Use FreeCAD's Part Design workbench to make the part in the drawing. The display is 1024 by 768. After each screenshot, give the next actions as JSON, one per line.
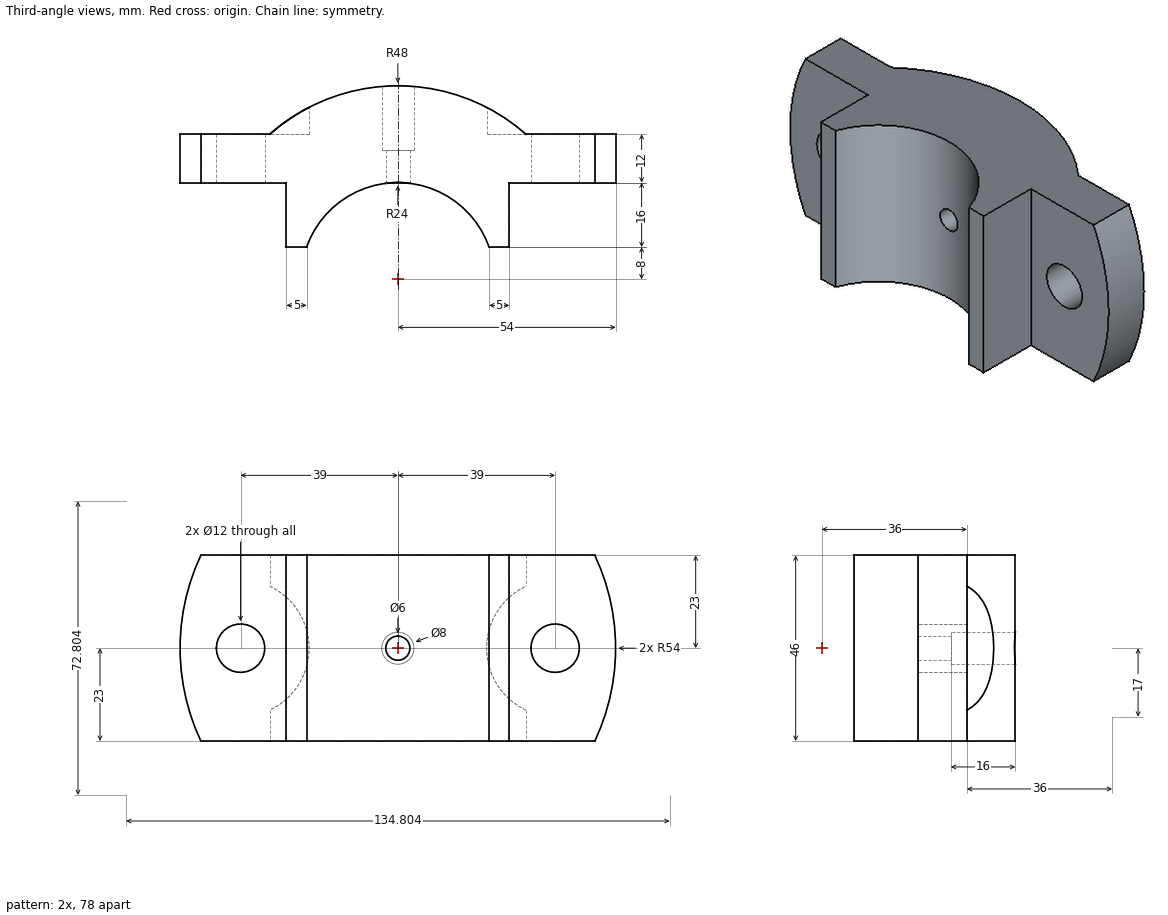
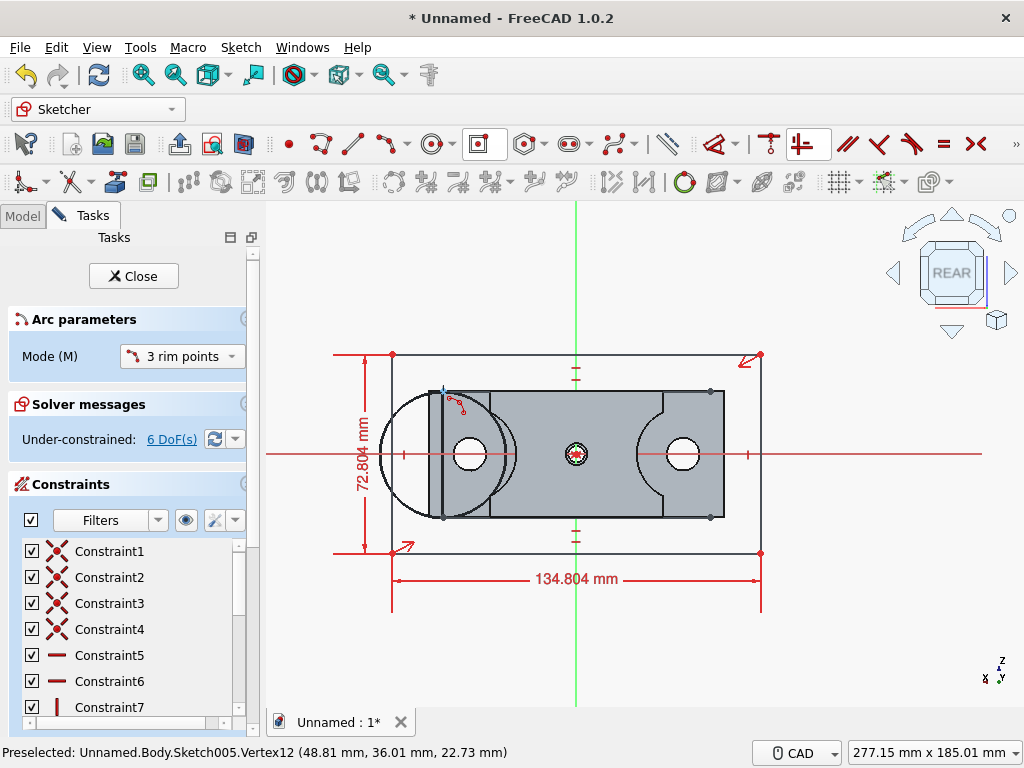
{"action": "scroll", "coordinate": [429, 441], "scroll_direction": "up", "scroll_amount": 2}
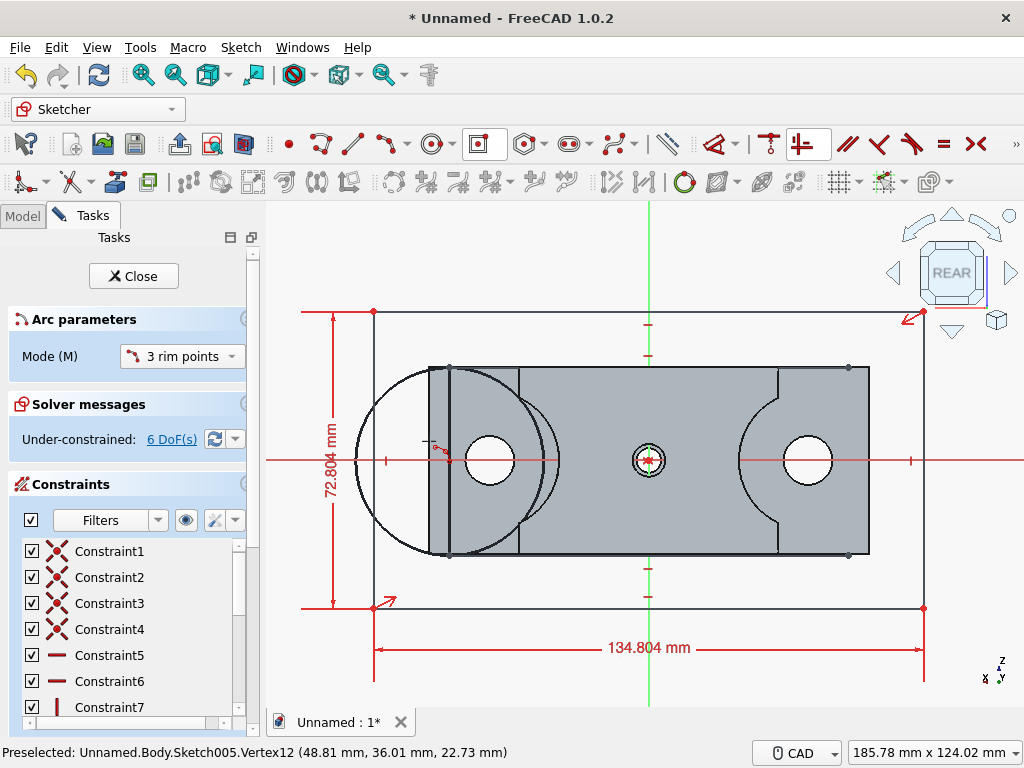
{"action": "left_click", "coordinate": [429, 441]}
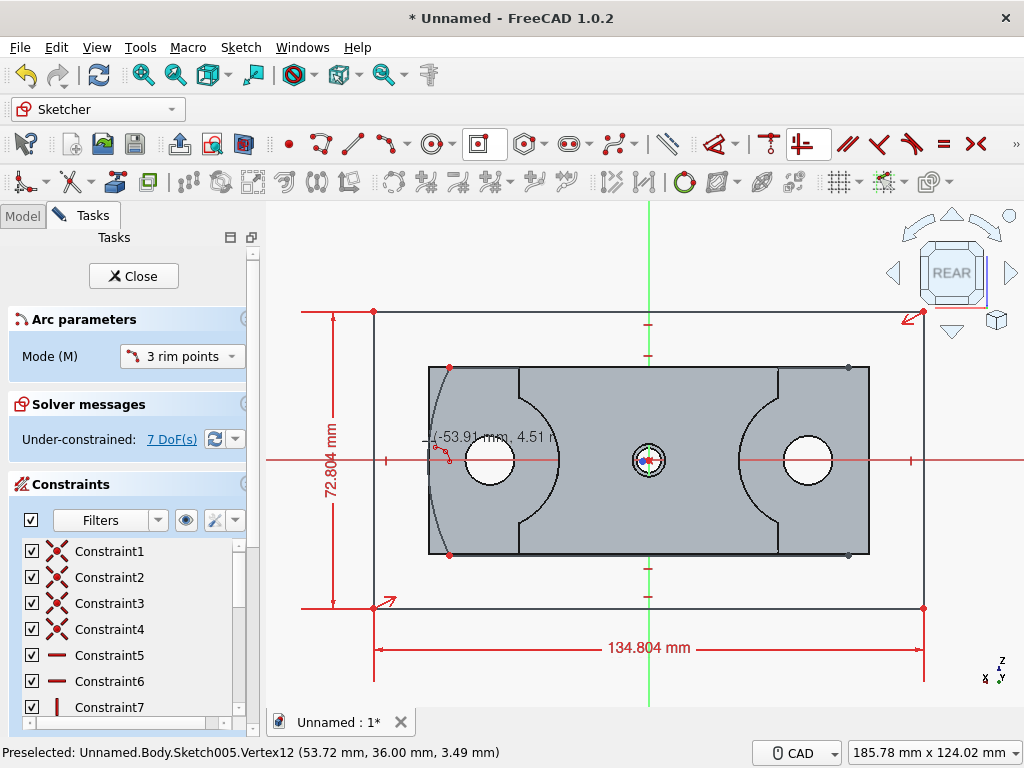
{"action": "left_click", "coordinate": [848, 368]}
{"action": "left_click", "coordinate": [848, 556]}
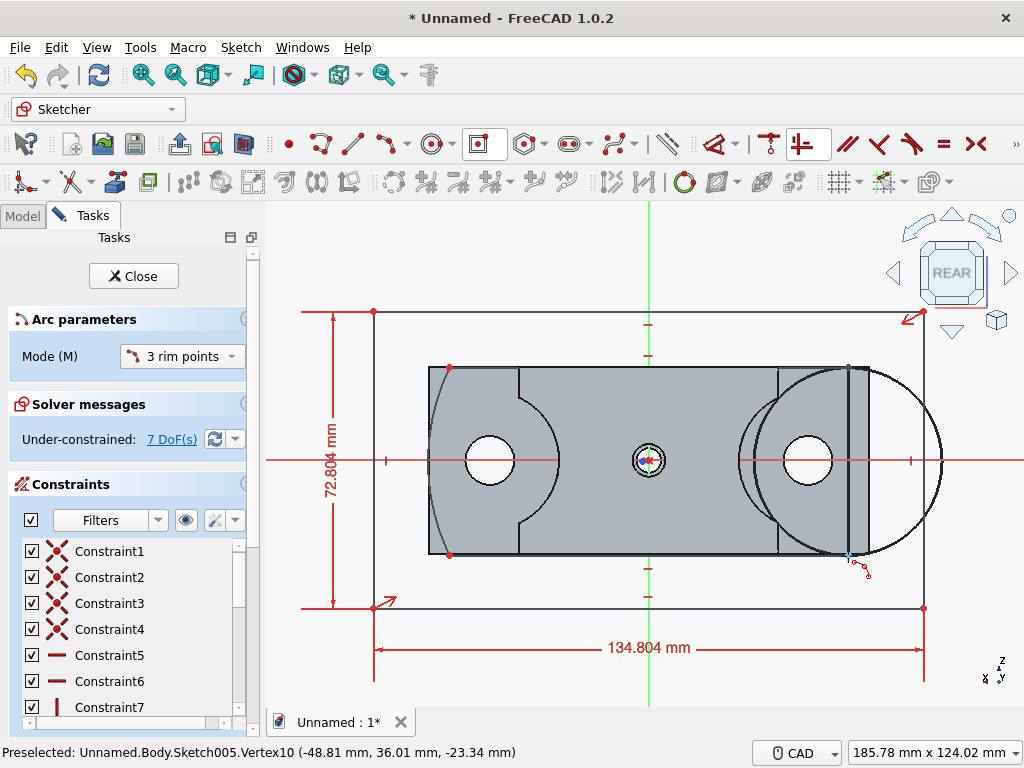
{"action": "scroll", "coordinate": [429, 441], "scroll_direction": "down", "scroll_amount": 2}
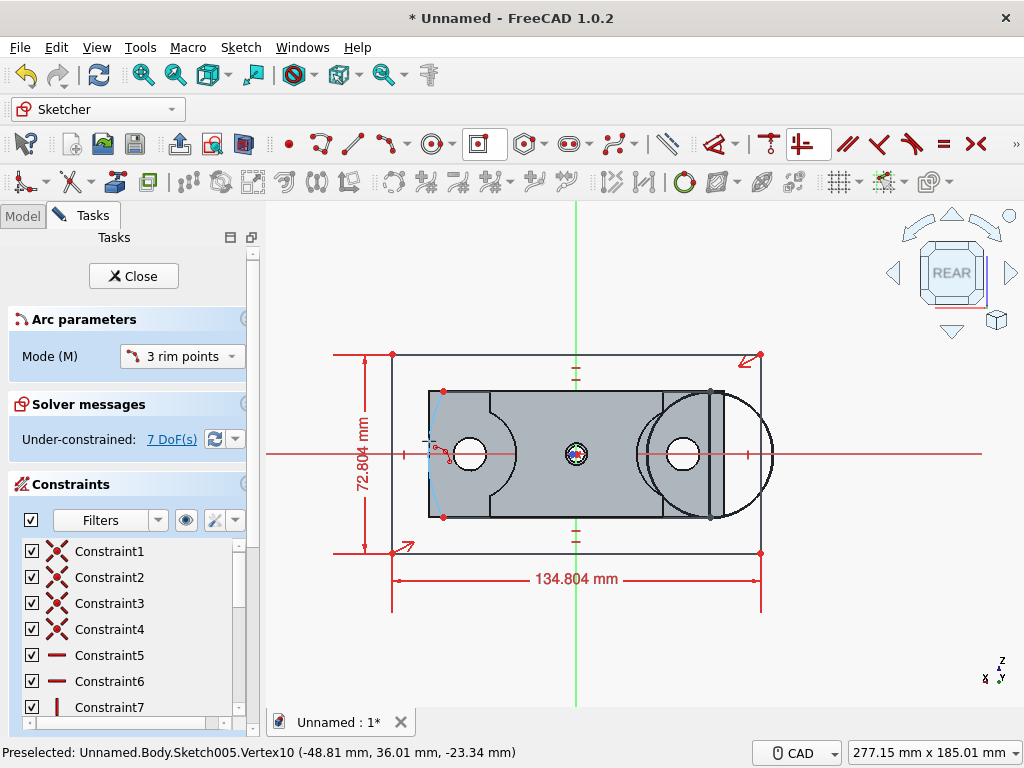
{"action": "scroll", "coordinate": [724, 467], "scroll_direction": "up", "scroll_amount": 2}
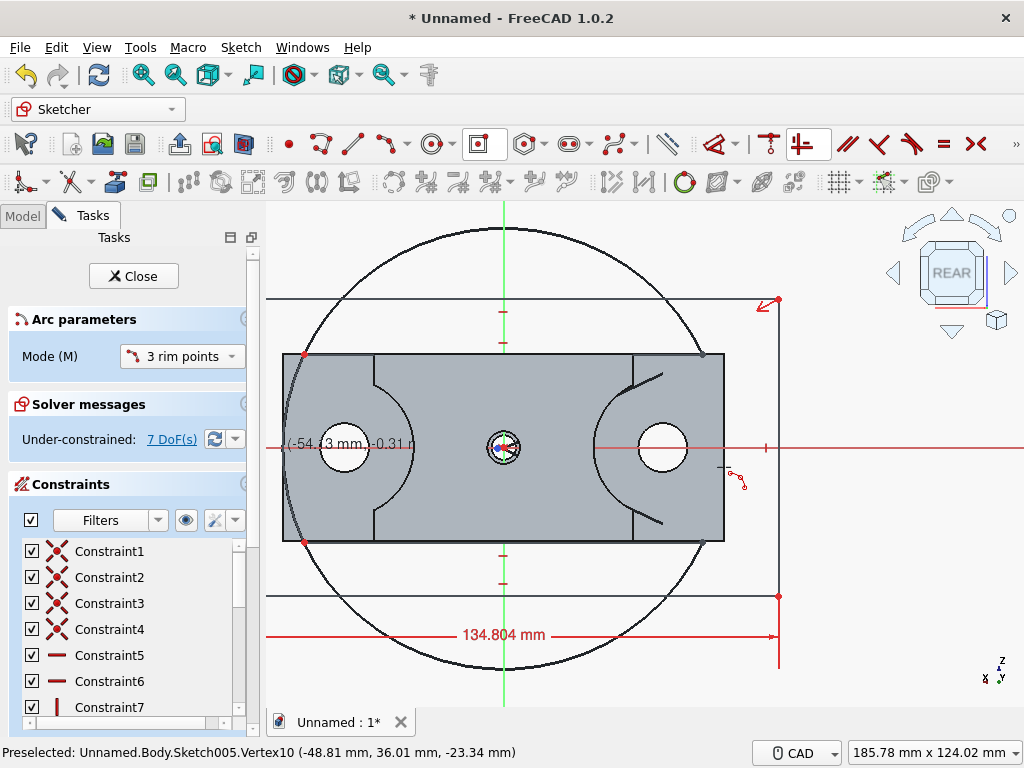
{"action": "left_click", "coordinate": [723, 467]}
{"action": "key", "text": "Escape"}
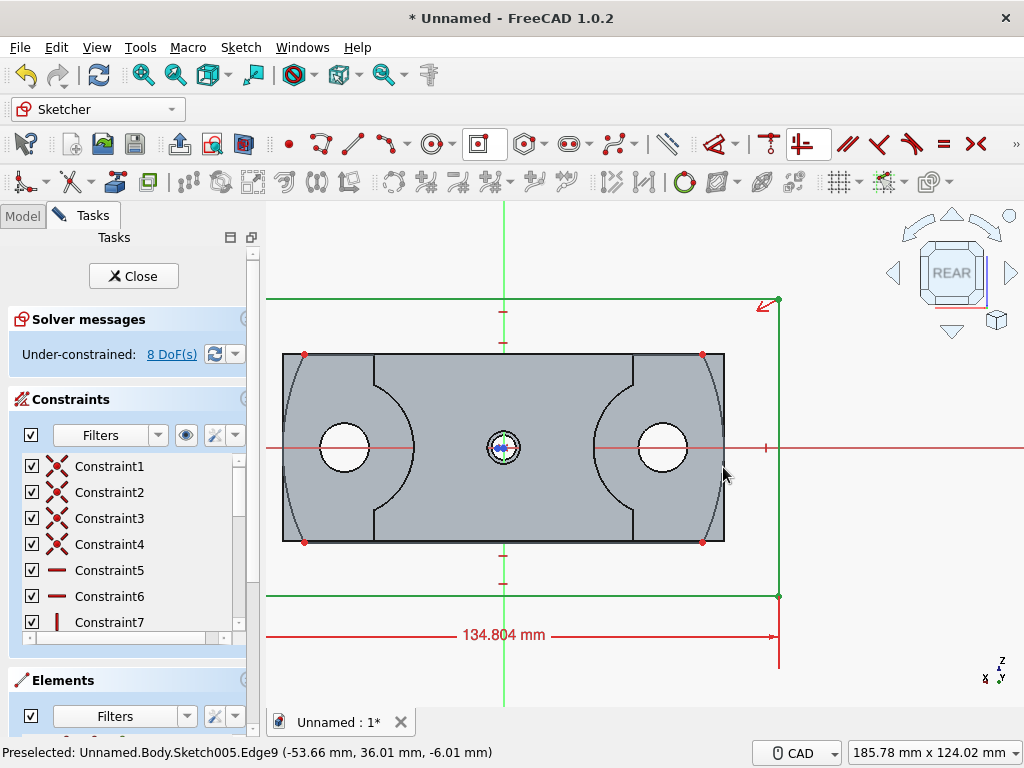
{"action": "scroll", "coordinate": [725, 467], "scroll_direction": "down", "scroll_amount": 2}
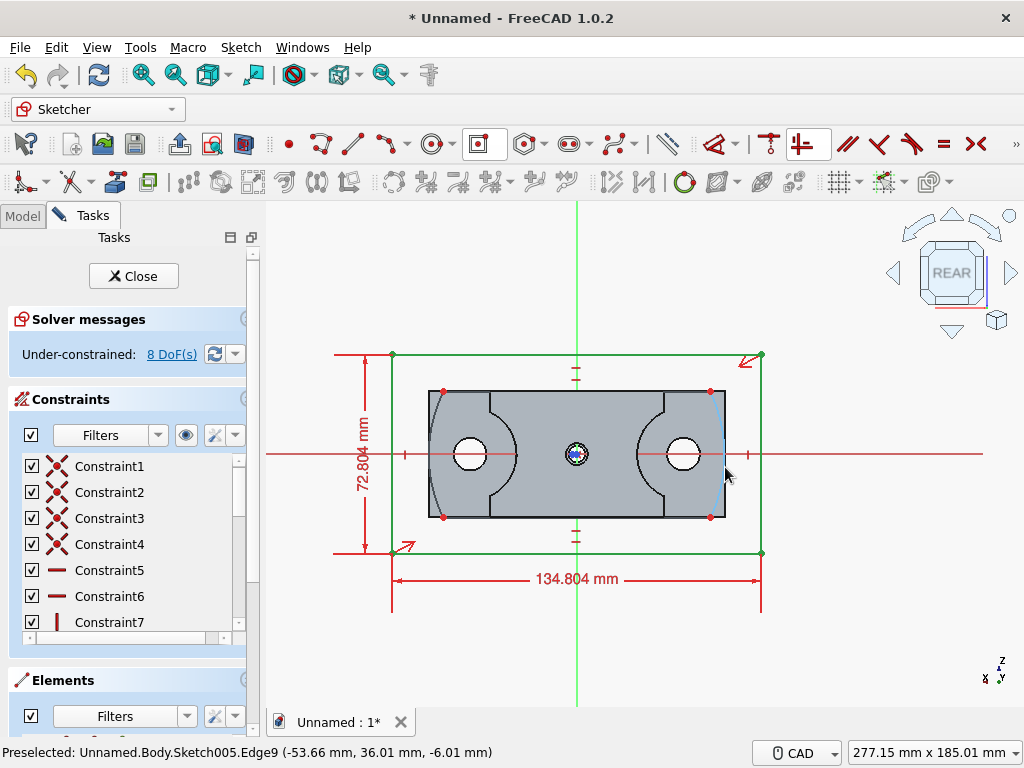
{"action": "left_click", "coordinate": [431, 429]}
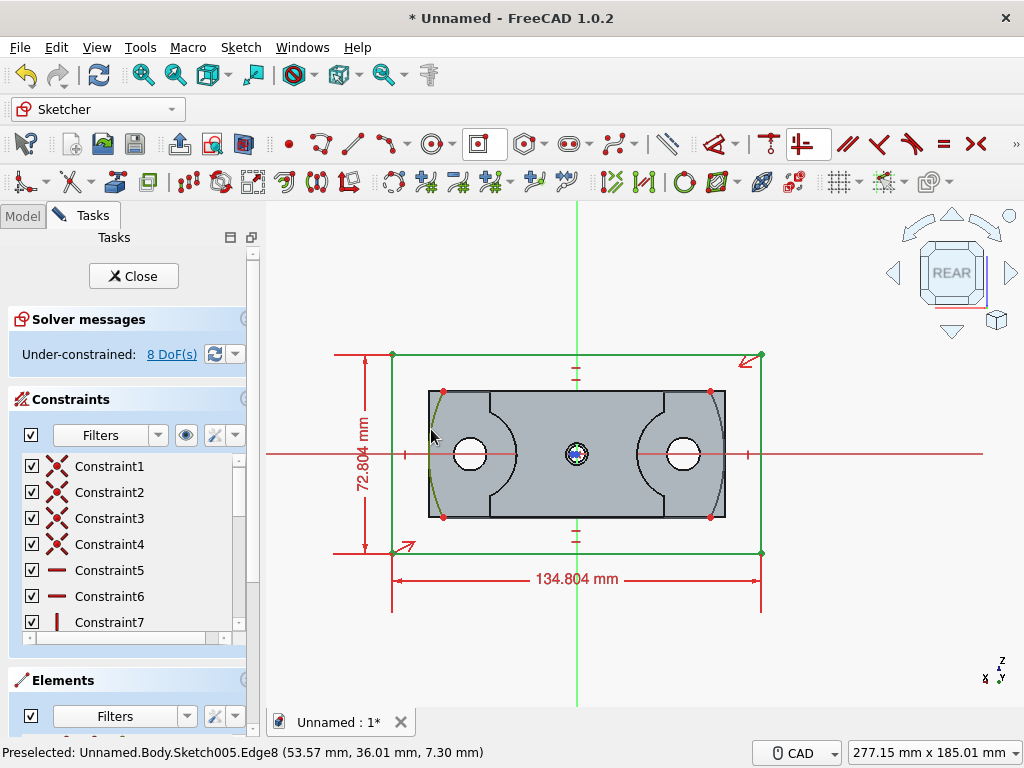
{"action": "left_click", "coordinate": [722, 481]}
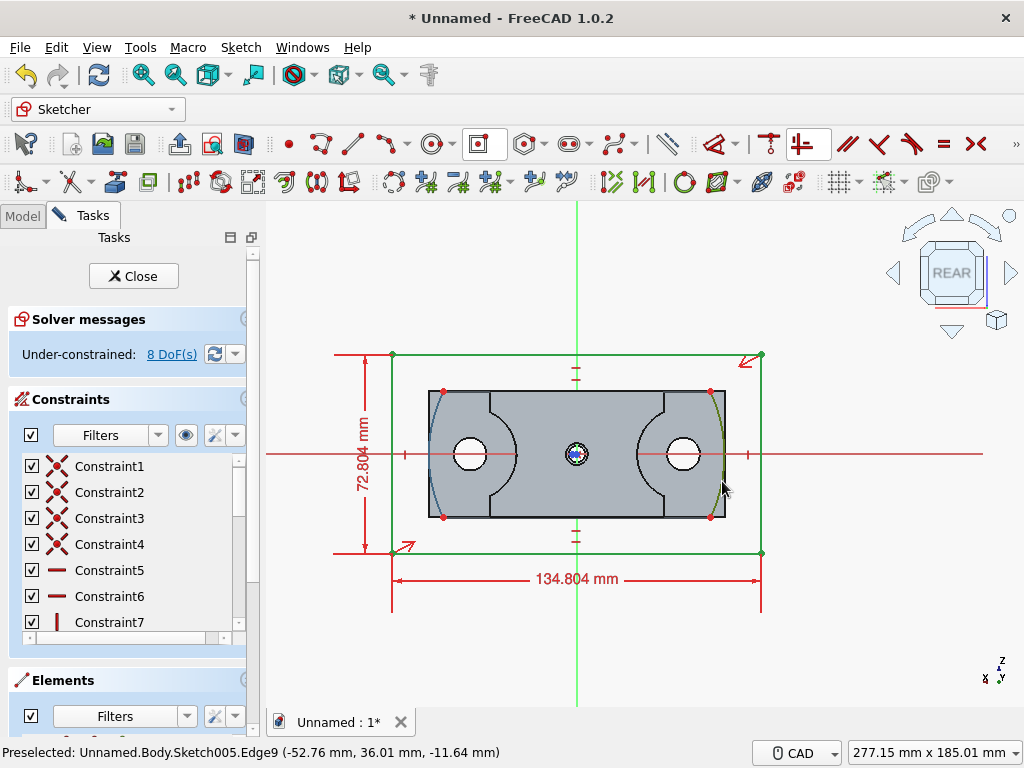
{"action": "left_click", "coordinate": [770, 144]}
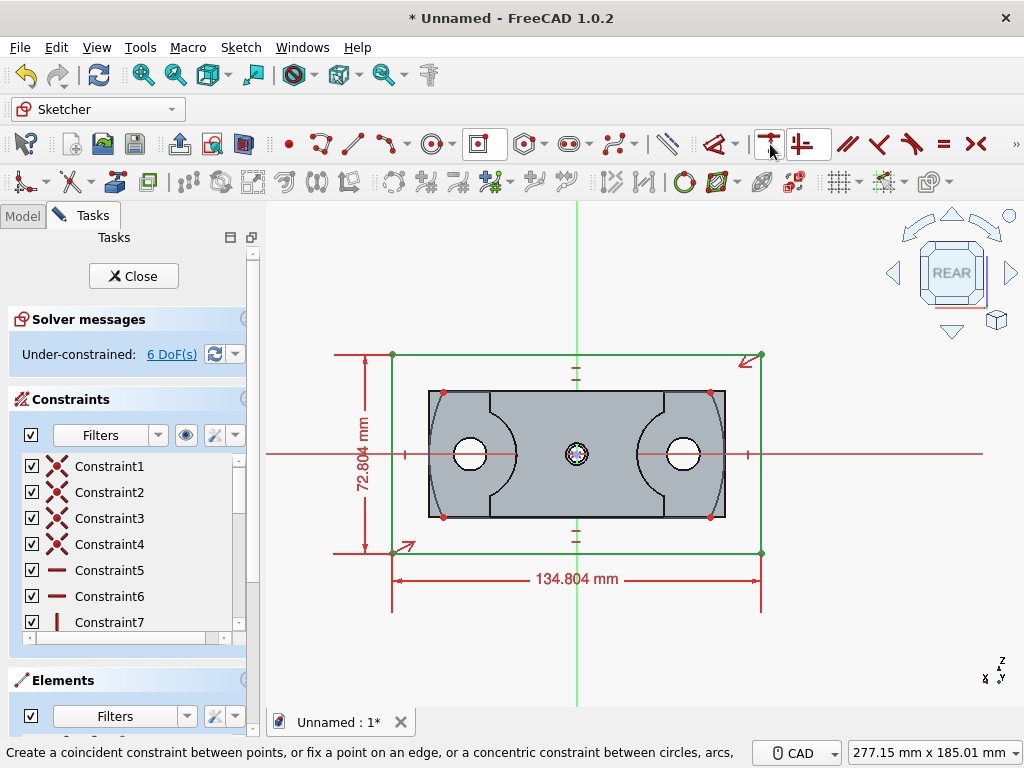
{"action": "left_click_drag", "start_coordinate": [566, 444], "coordinate": [587, 465]}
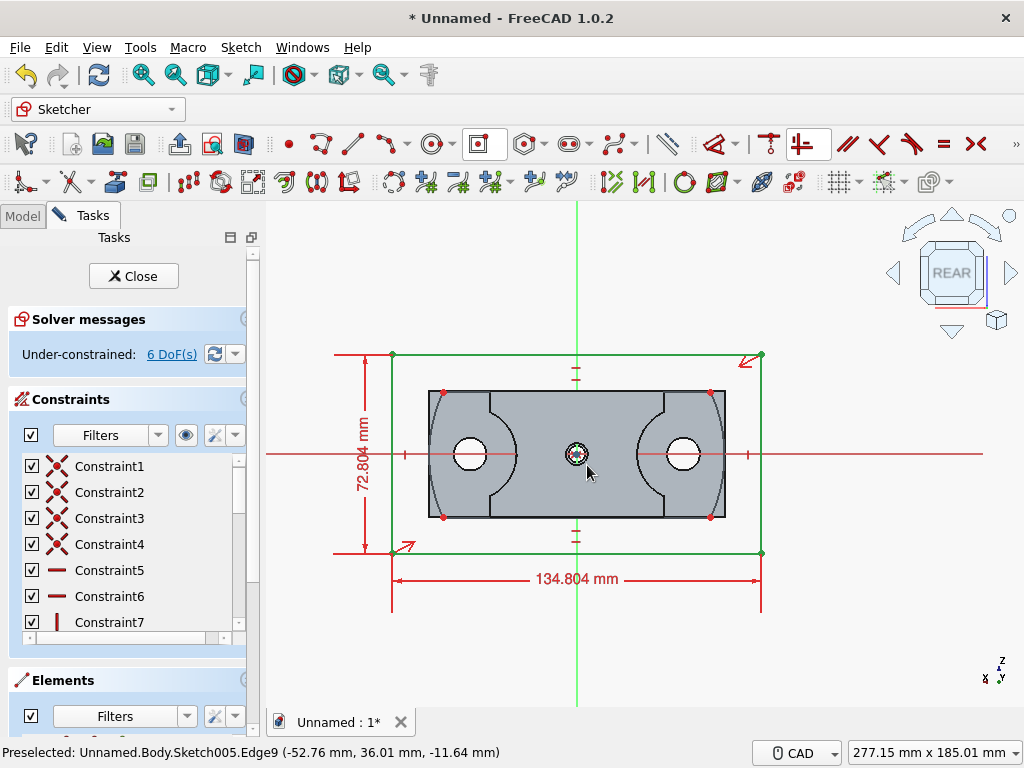
{"action": "left_click", "coordinate": [770, 144]}